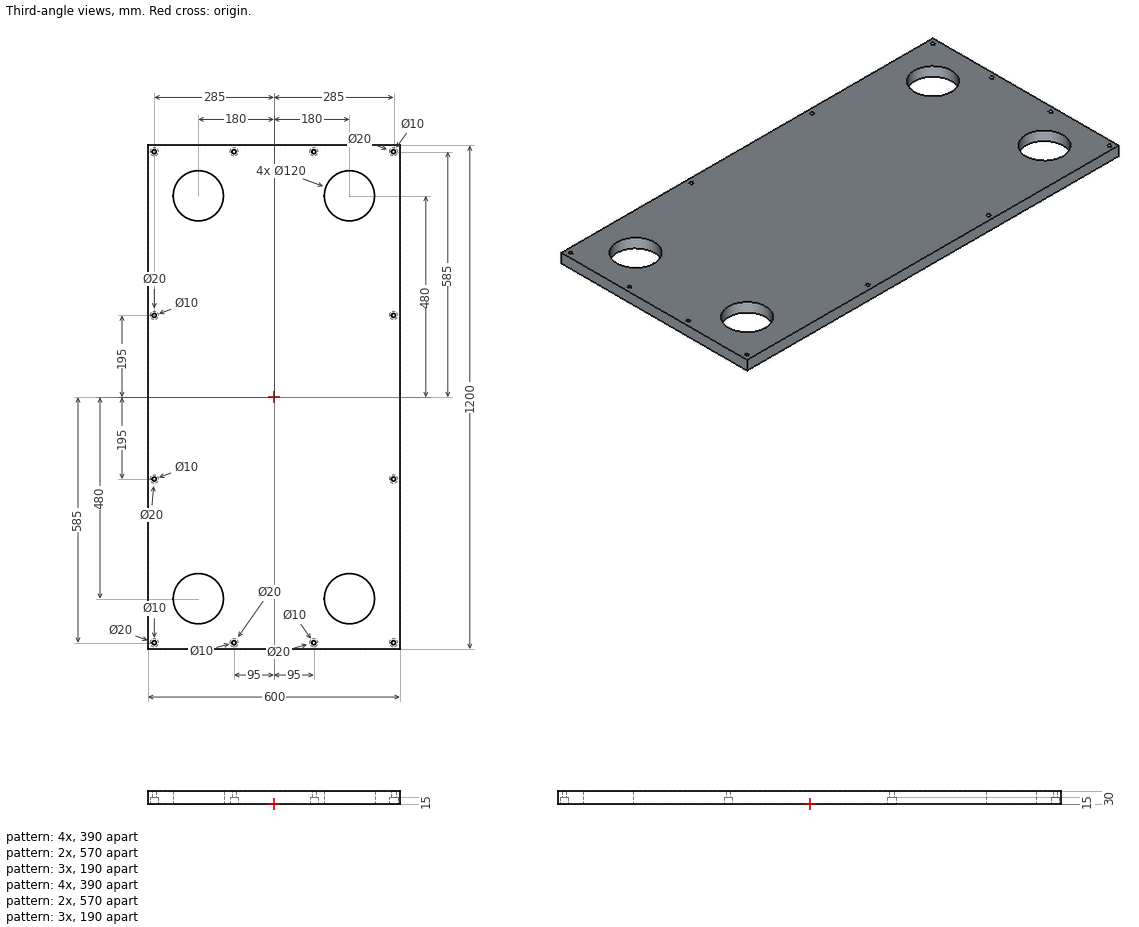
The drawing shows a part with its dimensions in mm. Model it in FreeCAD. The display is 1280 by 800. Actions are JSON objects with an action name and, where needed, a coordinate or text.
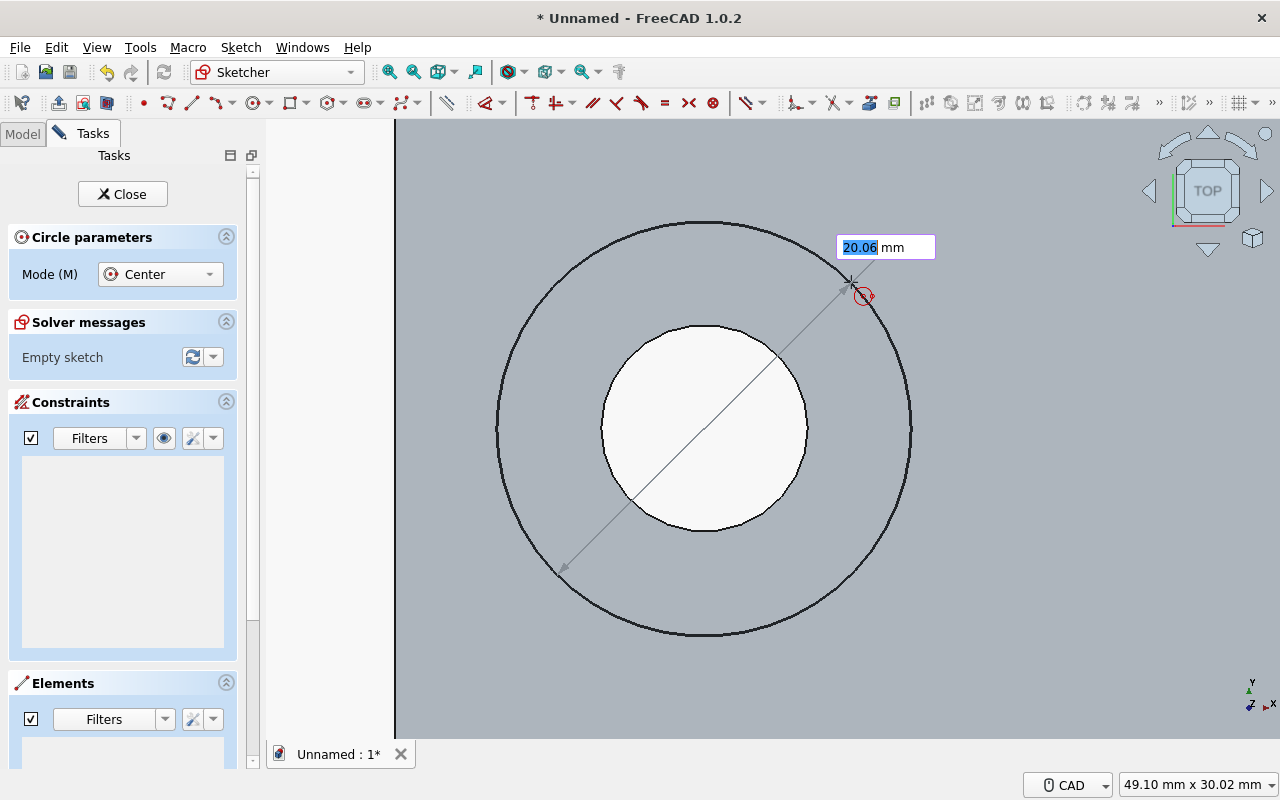
{"action": "type", "text": "20"}
{"action": "key", "text": "Return"}
{"action": "key", "text": "Escape"}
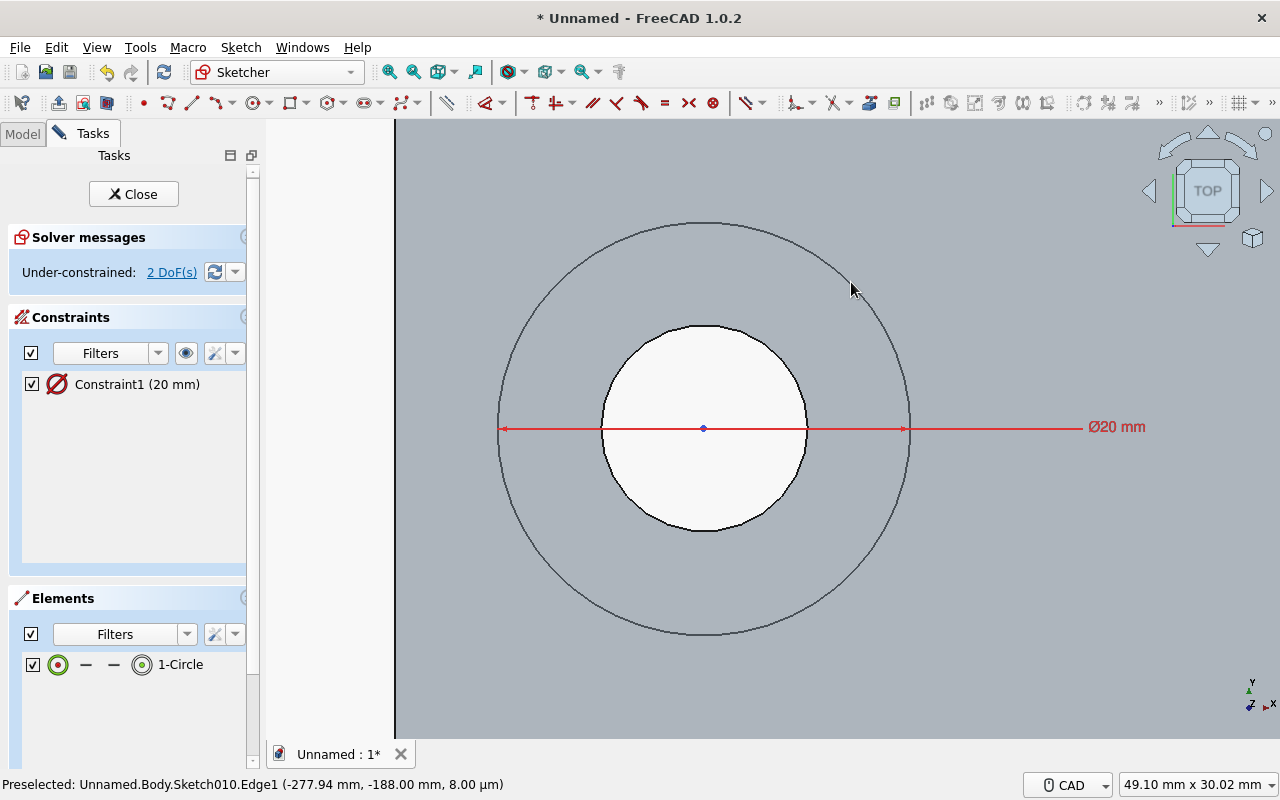
{"action": "key", "text": "d"}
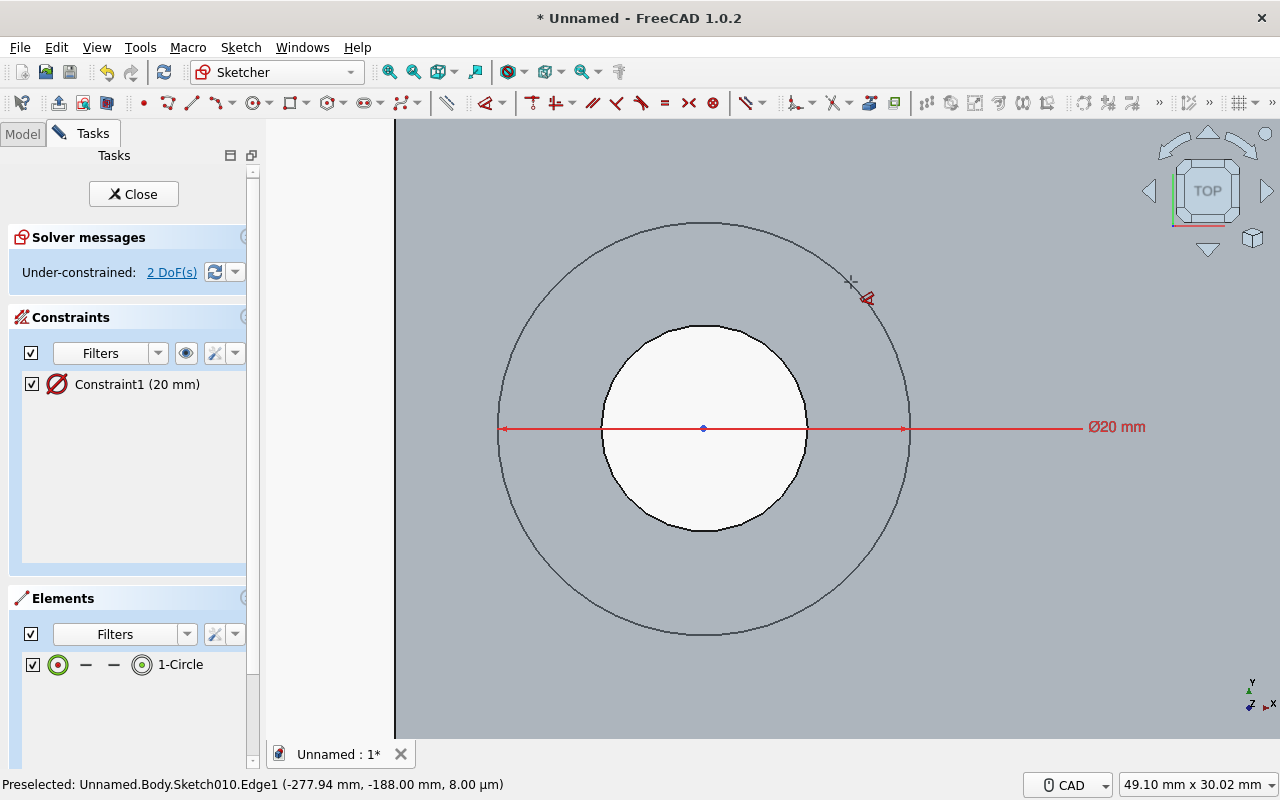
{"action": "left_click", "coordinate": [704, 429]}
{"action": "left_click", "coordinate": [815, 463]}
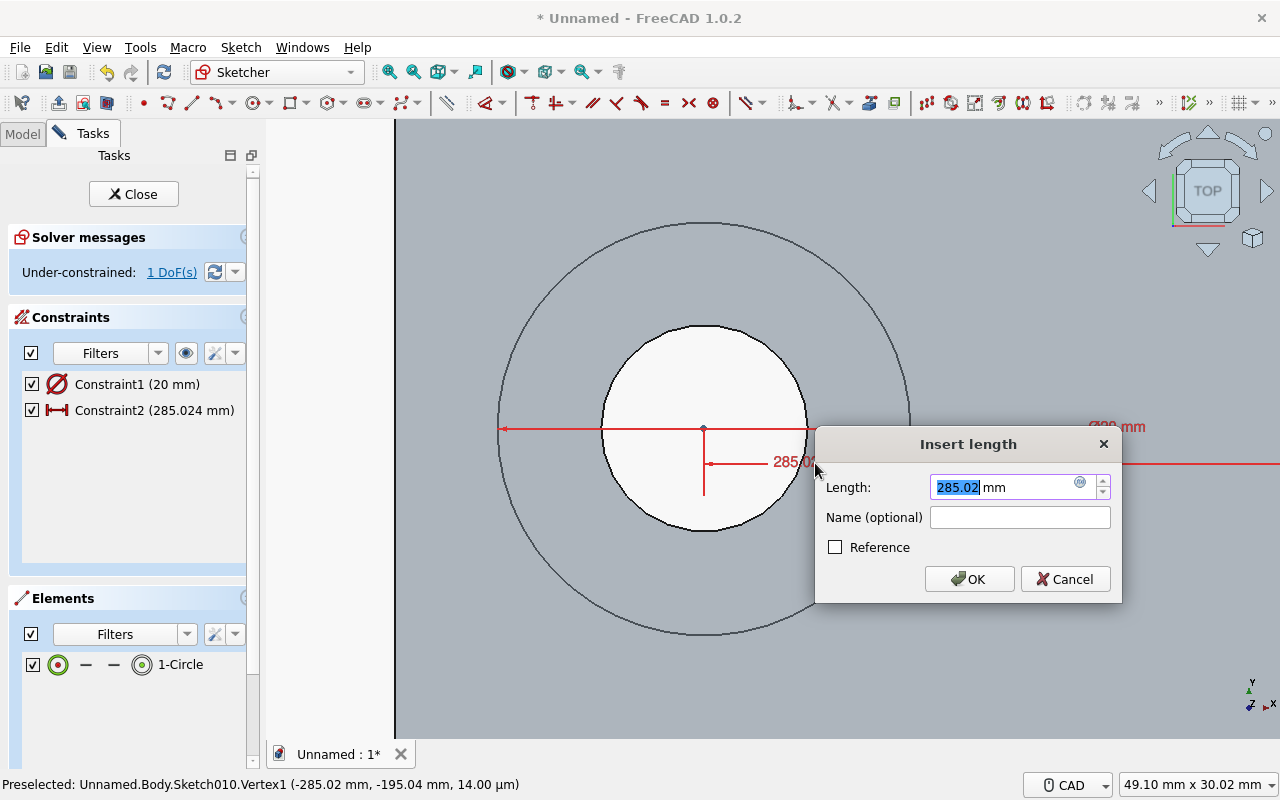
{"action": "type", "text": "285"}
{"action": "key", "text": "Return"}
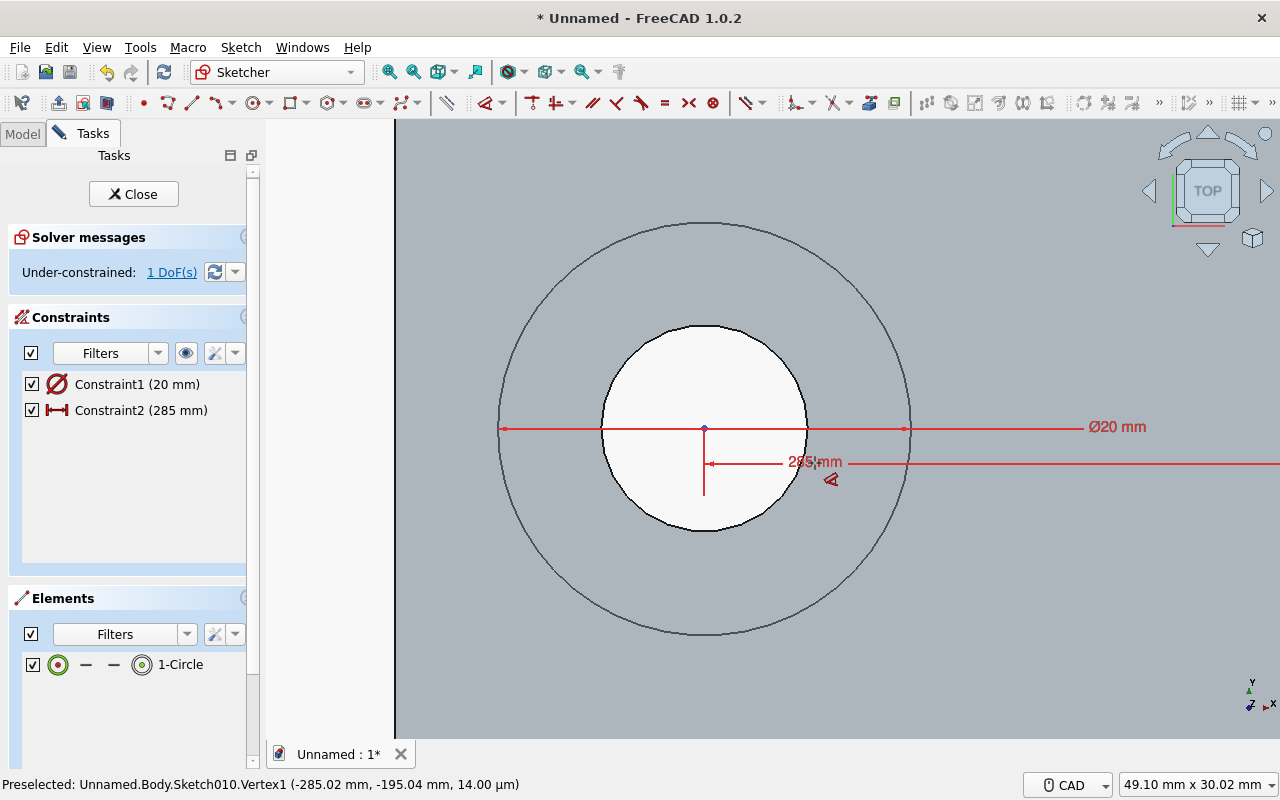
{"action": "left_click", "coordinate": [704, 429]}
{"action": "left_click", "coordinate": [670, 288]}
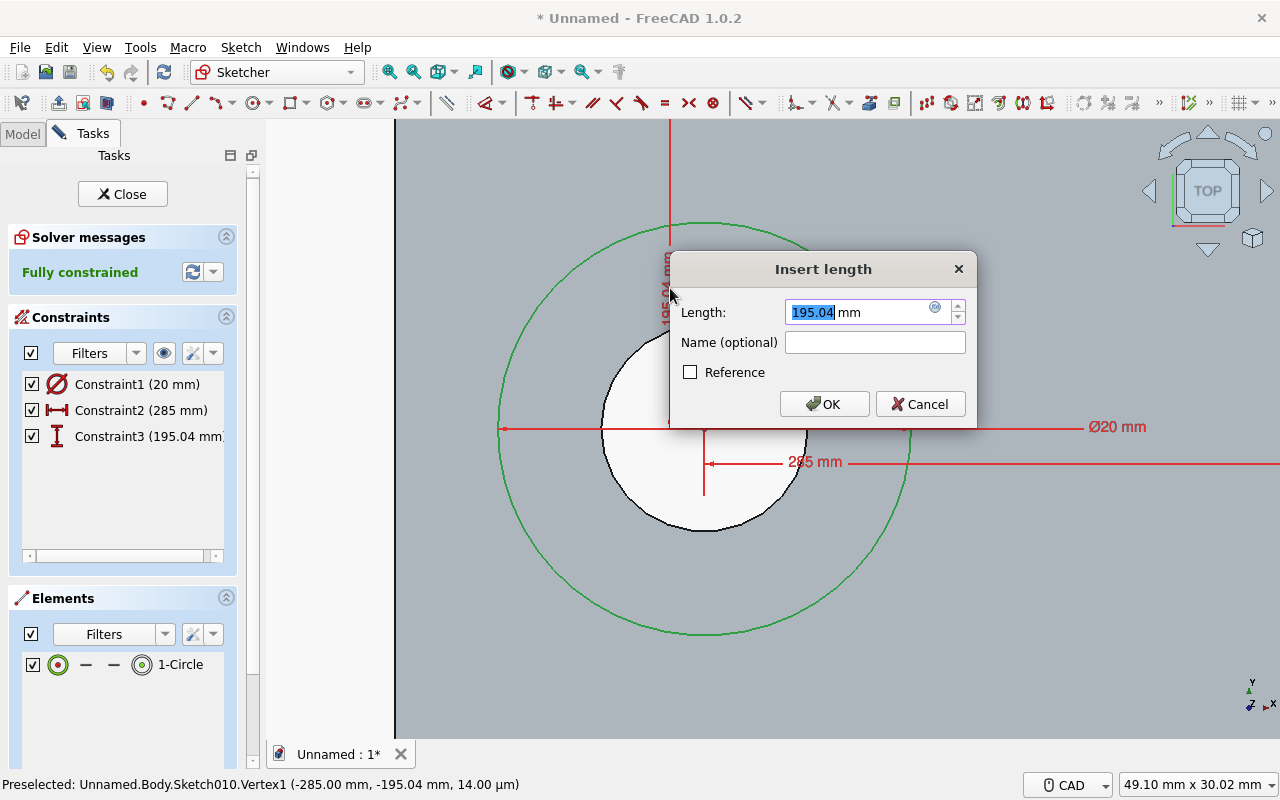
{"action": "type", "text": "195"}
{"action": "key", "text": "Return"}
{"action": "key", "text": "Escape"}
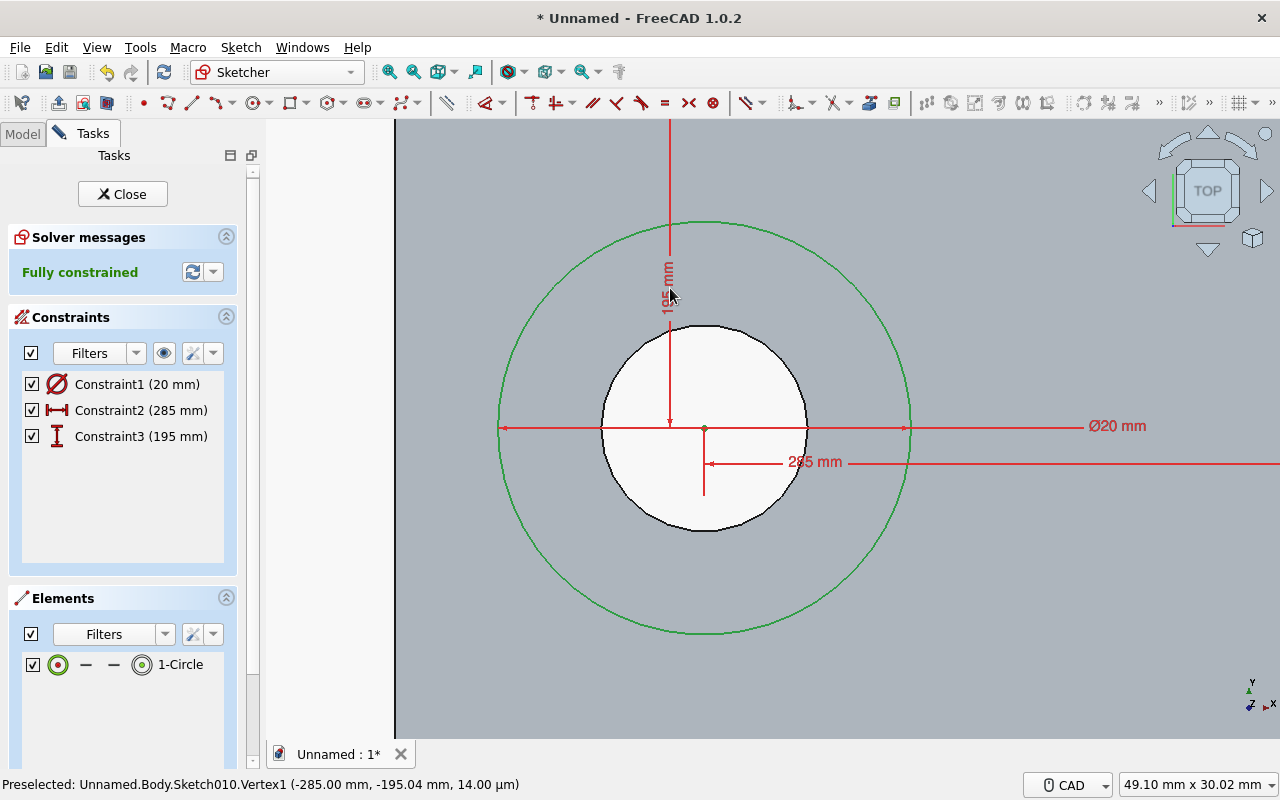
{"action": "left_click", "coordinate": [123, 194]}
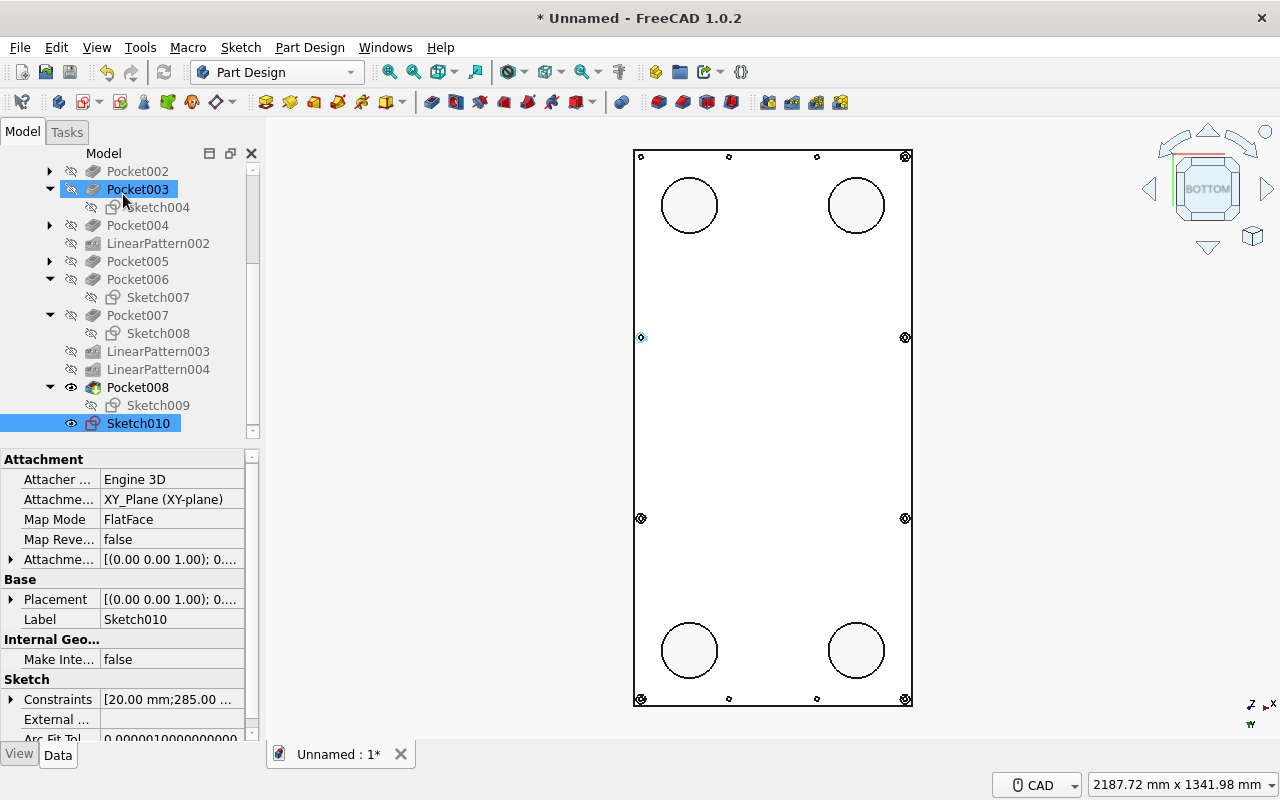
{"action": "left_click", "coordinate": [432, 102]}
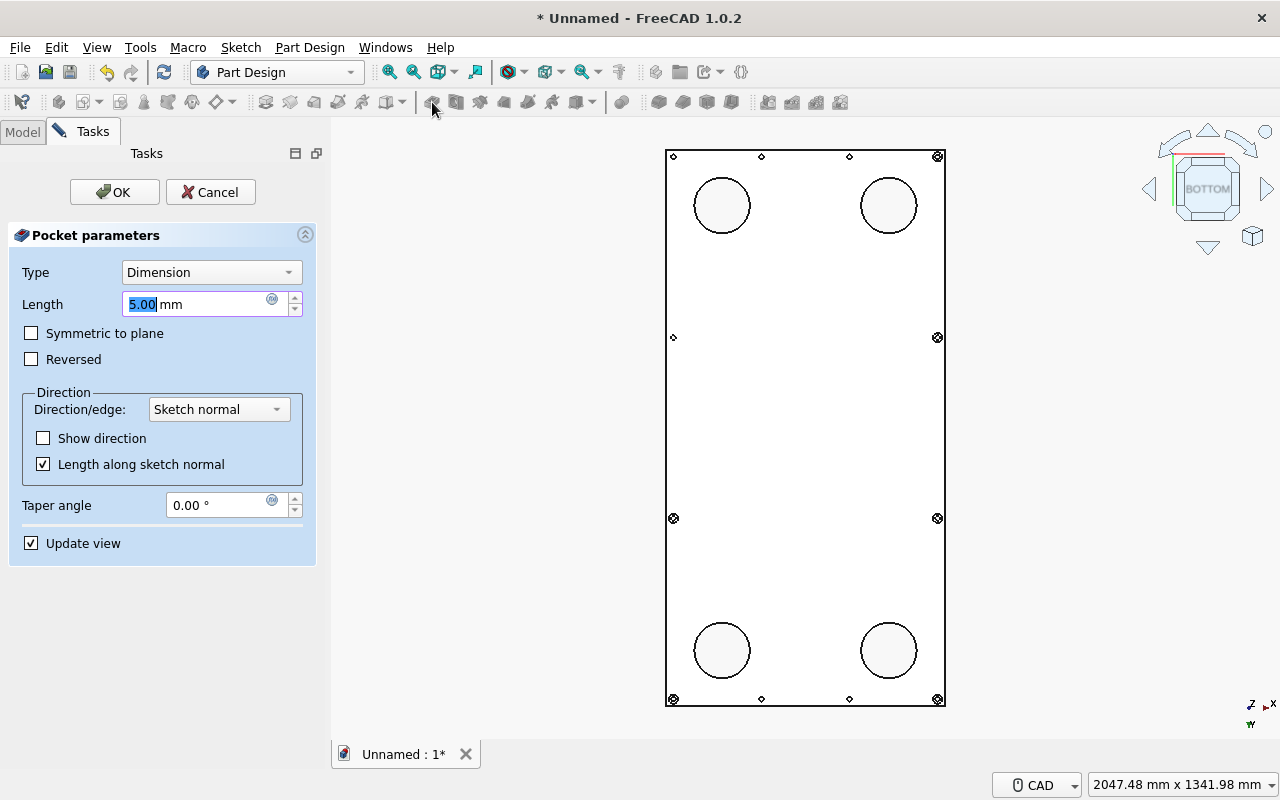
{"action": "type", "text": "15"}
{"action": "key", "text": "Tab"}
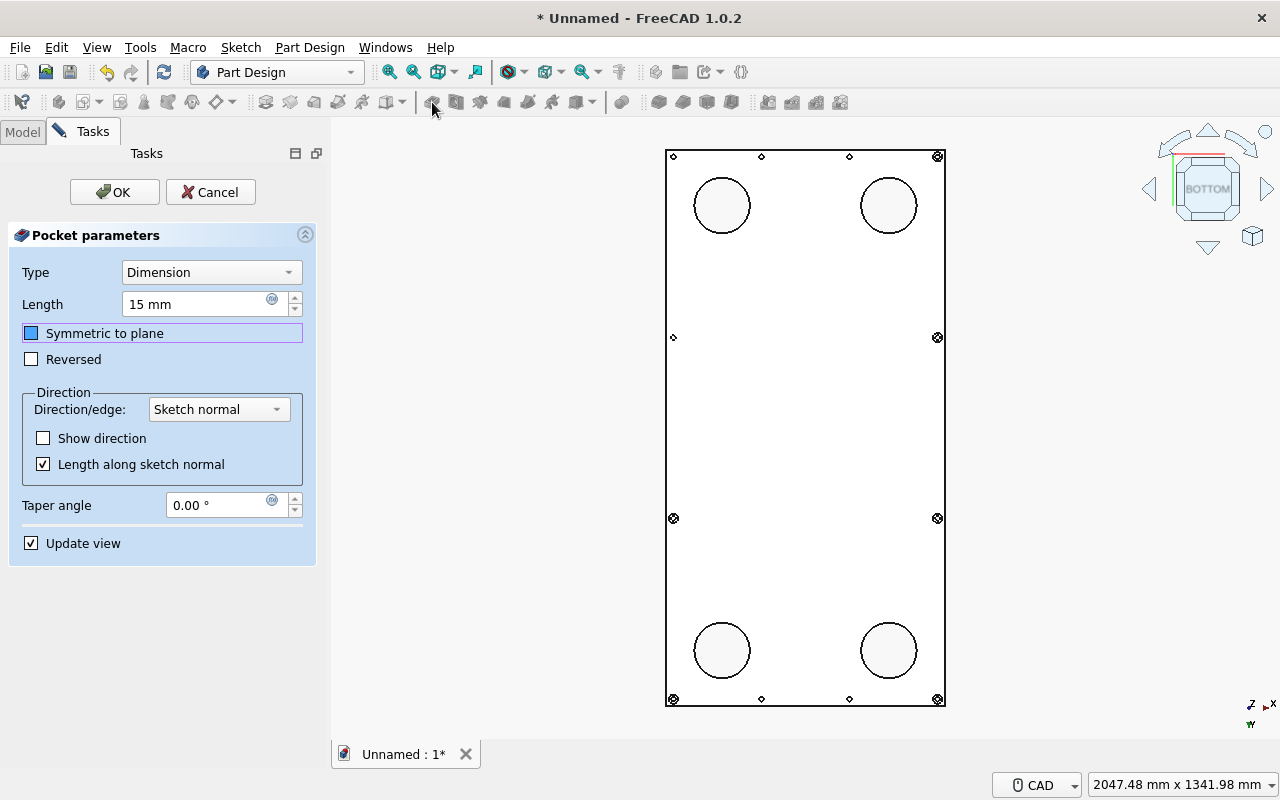
{"action": "left_click", "coordinate": [30, 359]}